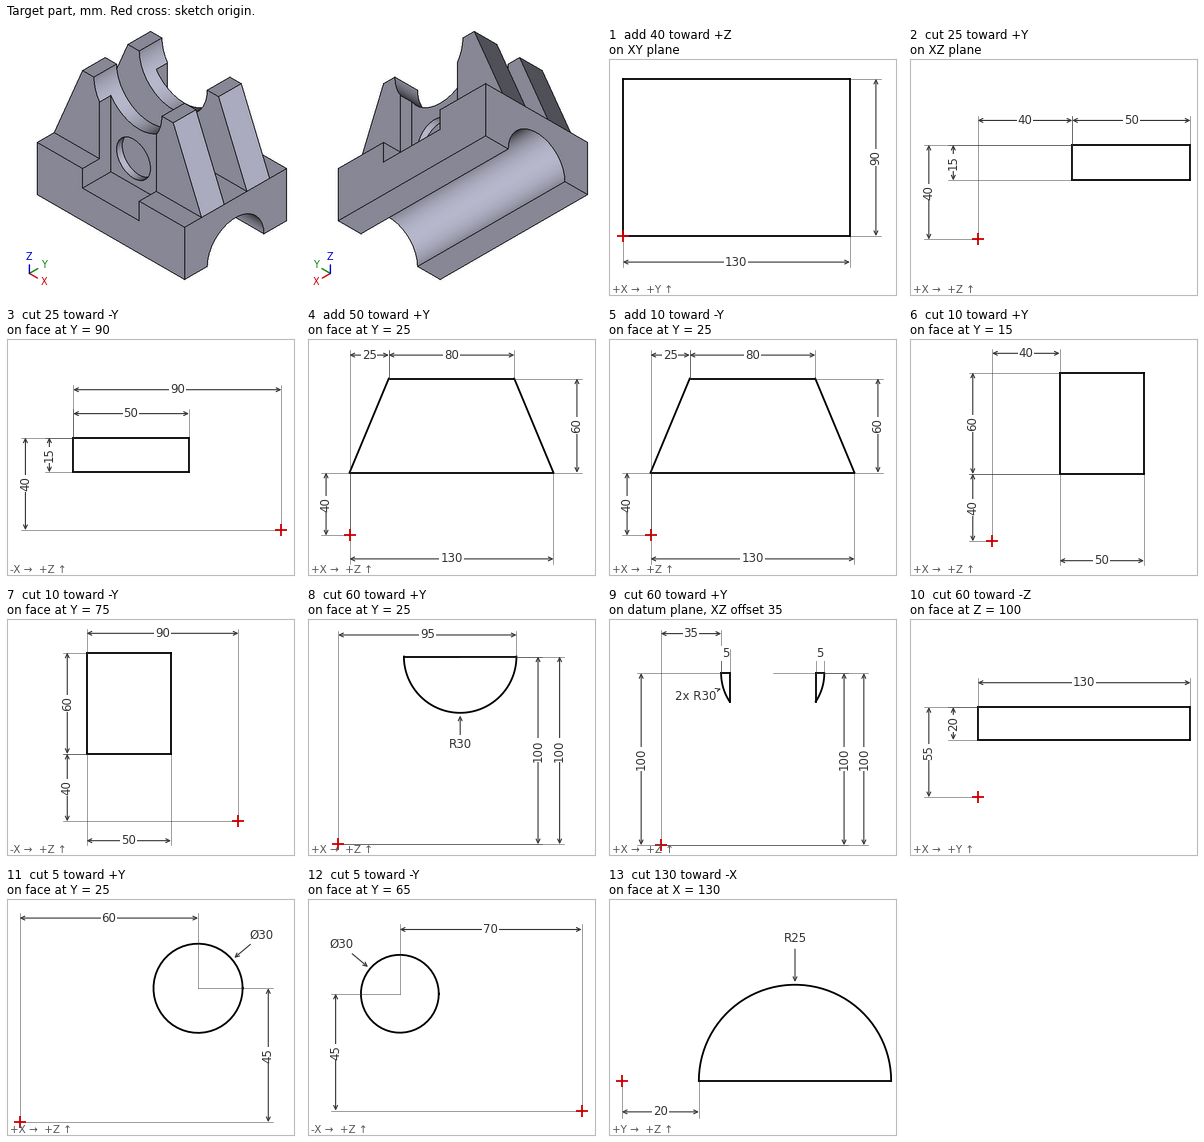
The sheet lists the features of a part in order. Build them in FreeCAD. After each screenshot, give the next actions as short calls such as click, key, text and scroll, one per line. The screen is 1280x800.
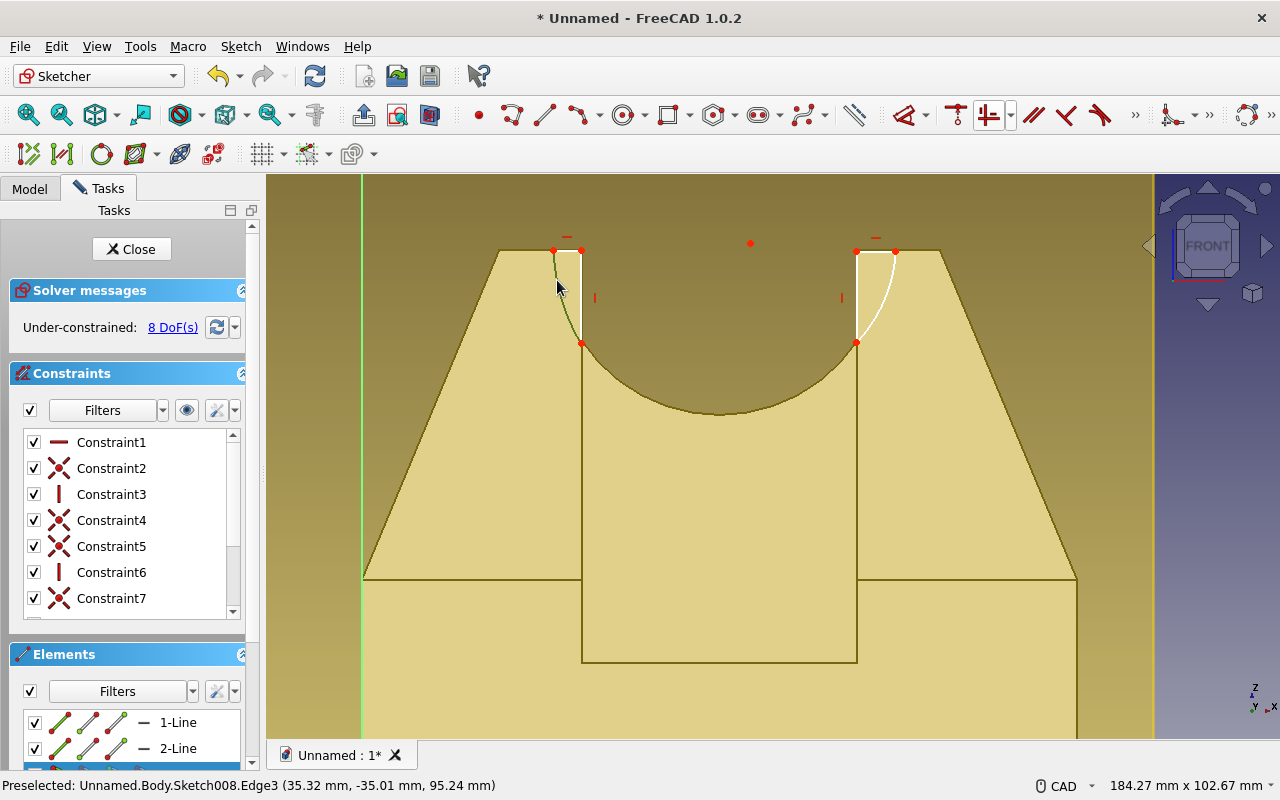
click(875, 319)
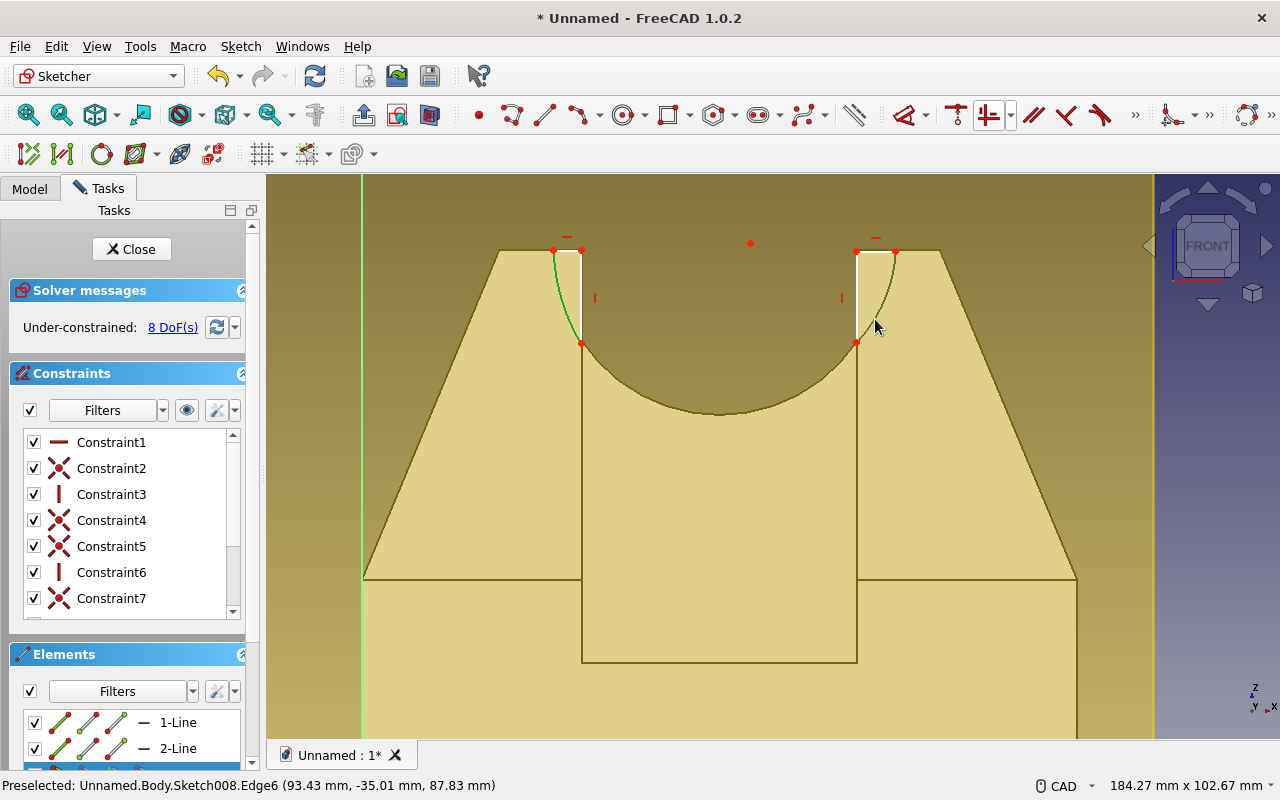
key(e)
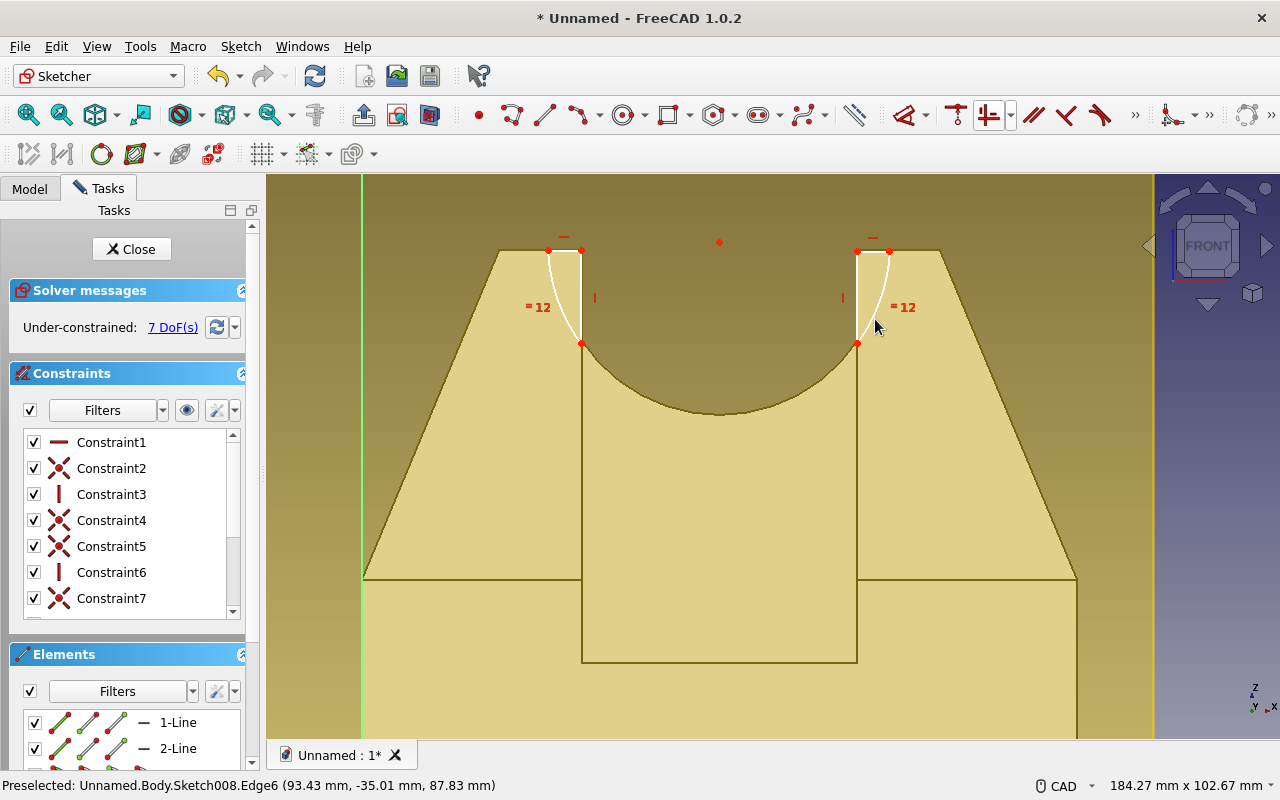
key(d)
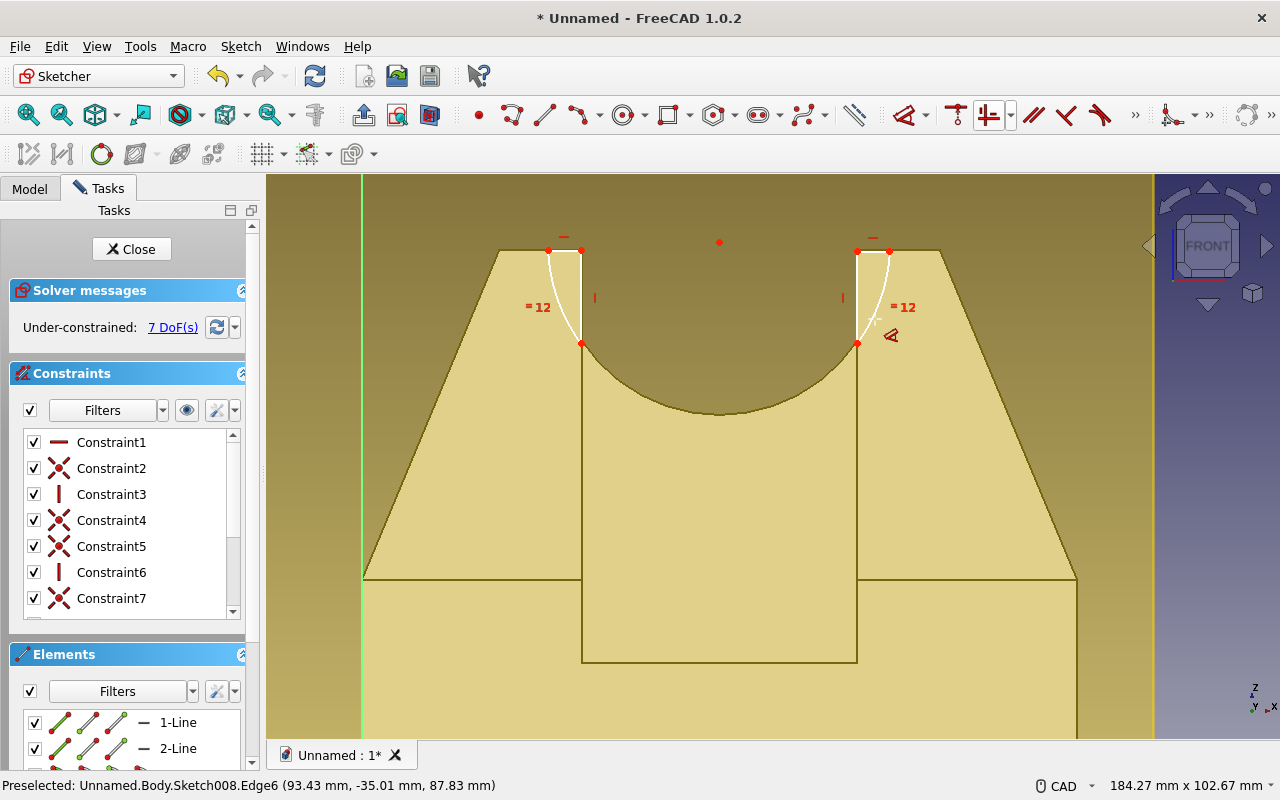
click(552, 280)
click(521, 287)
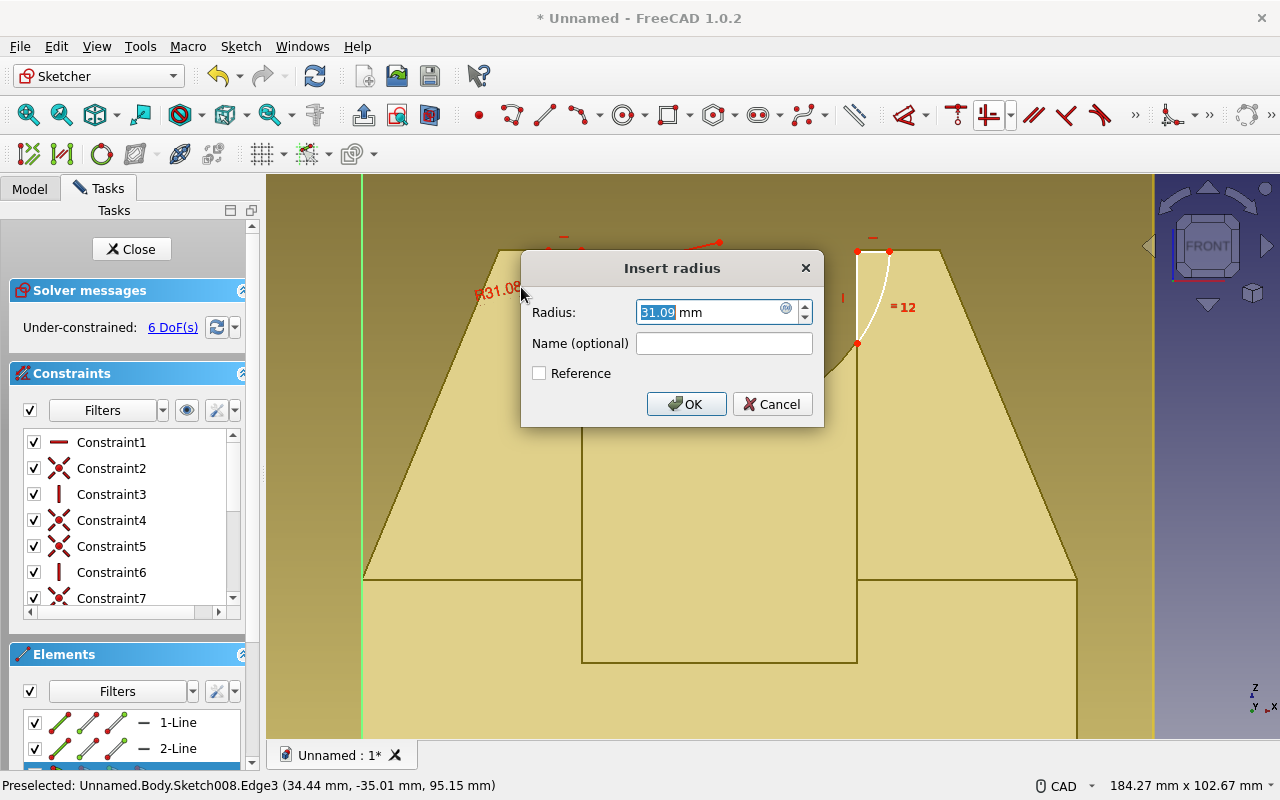
text(30)
key(Return)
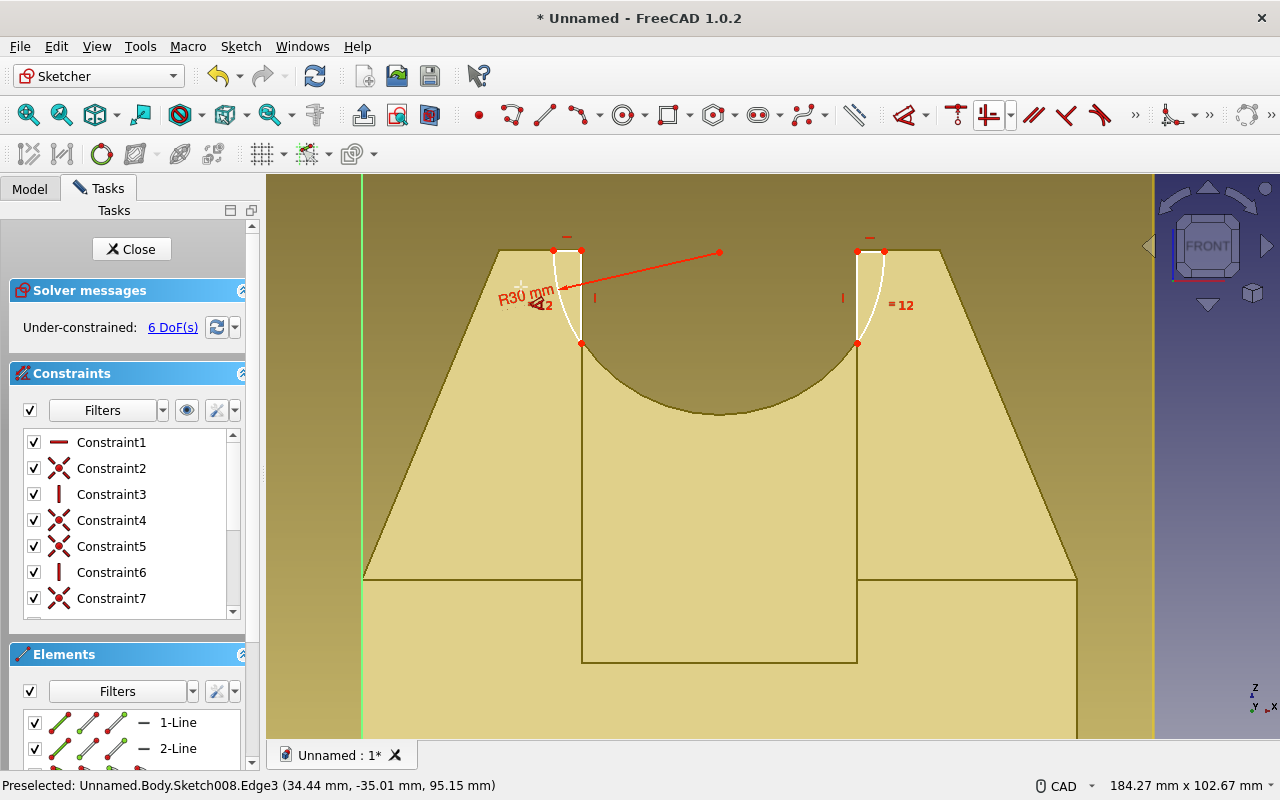
scroll(565, 251, up, 2)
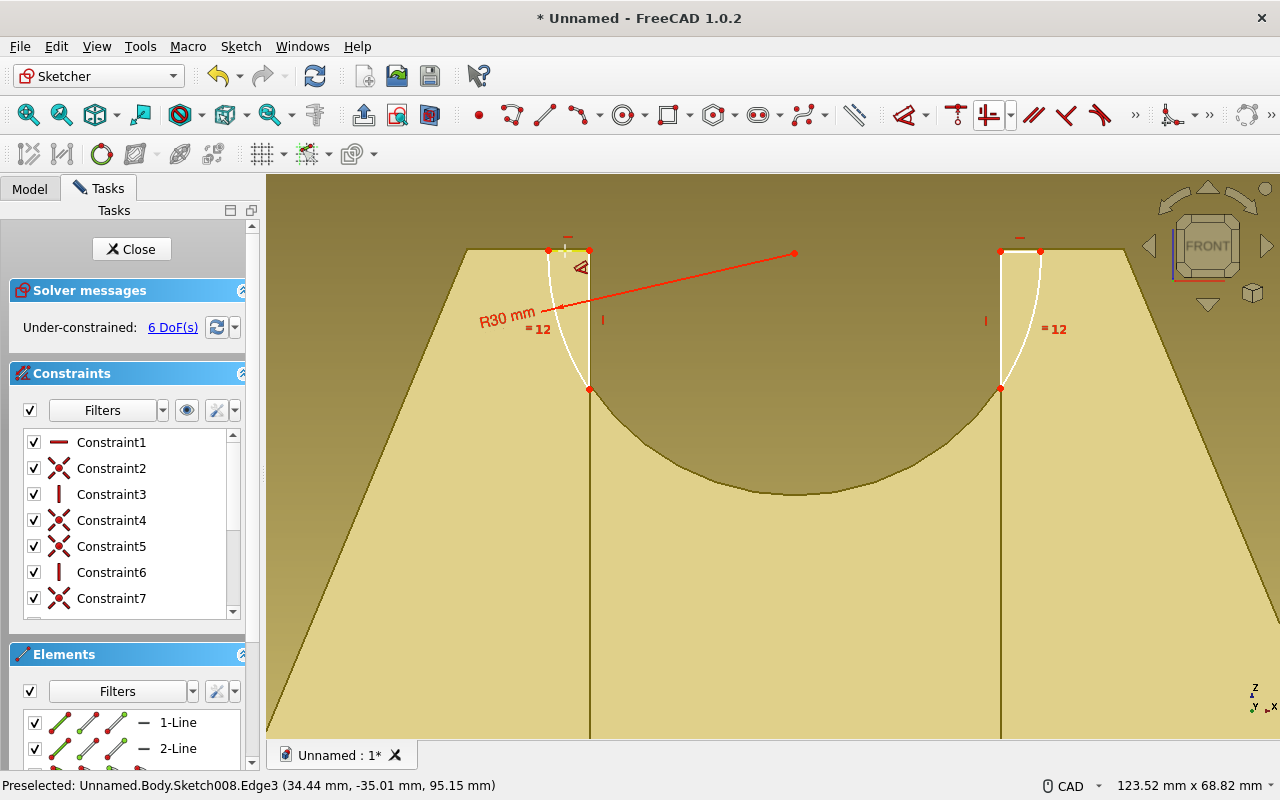
click(565, 251)
click(569, 217)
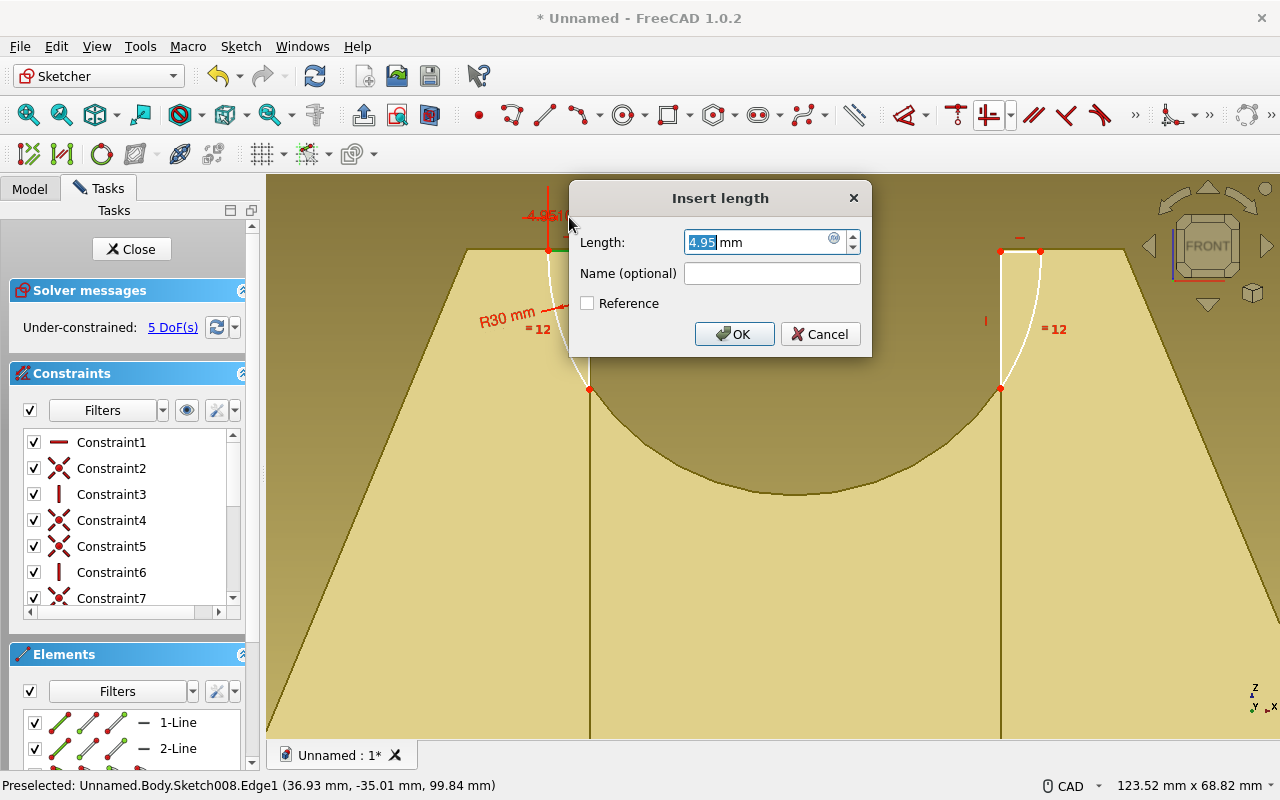
text(5)
key(Return)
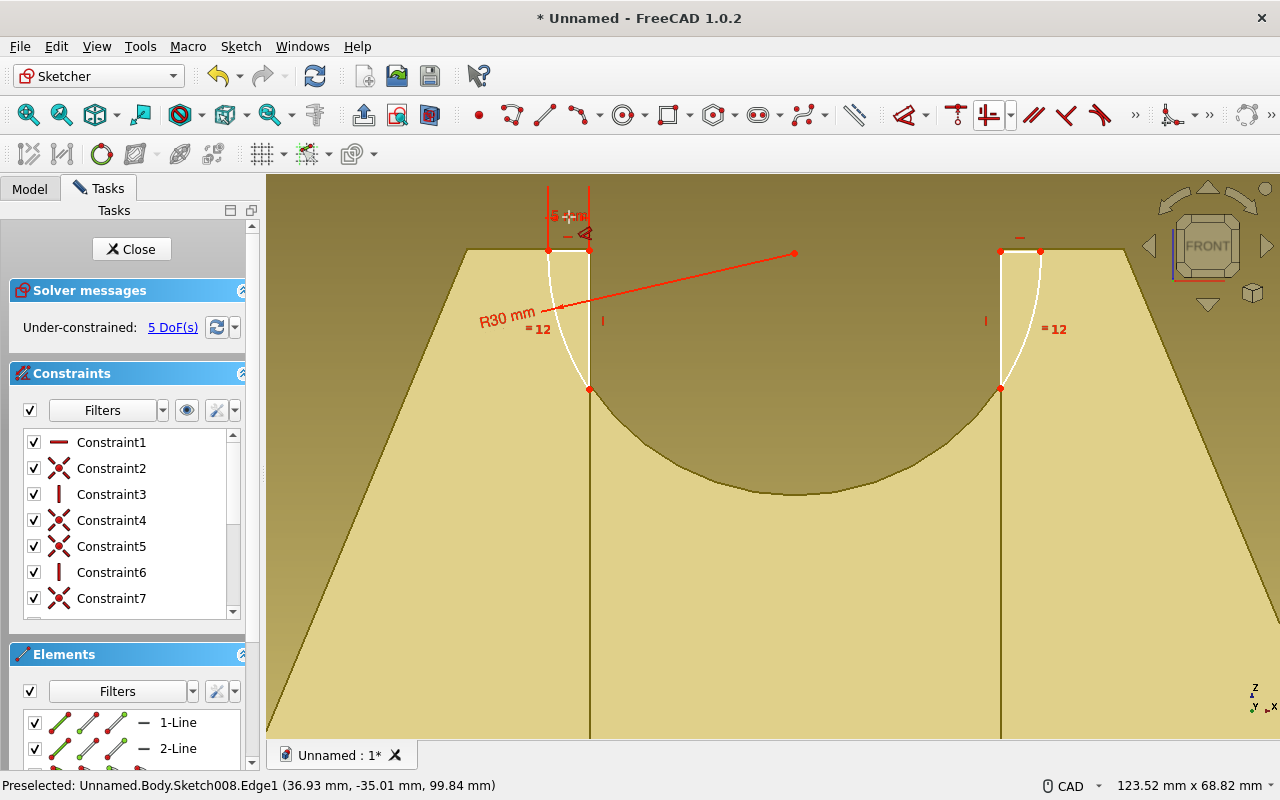
click(1013, 252)
click(1021, 218)